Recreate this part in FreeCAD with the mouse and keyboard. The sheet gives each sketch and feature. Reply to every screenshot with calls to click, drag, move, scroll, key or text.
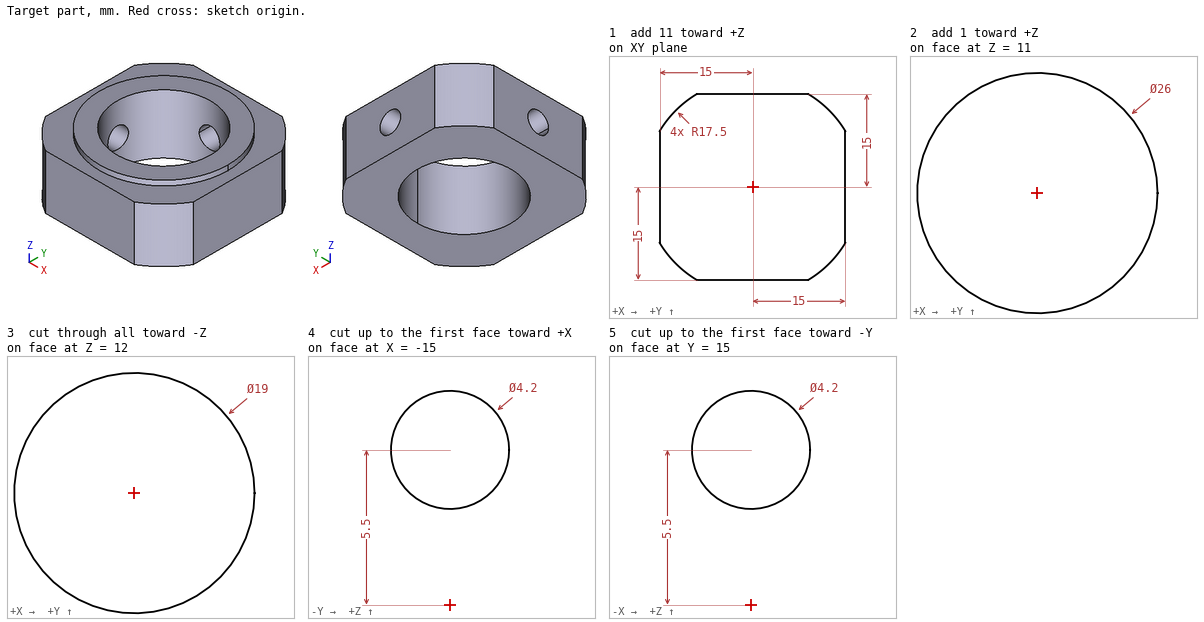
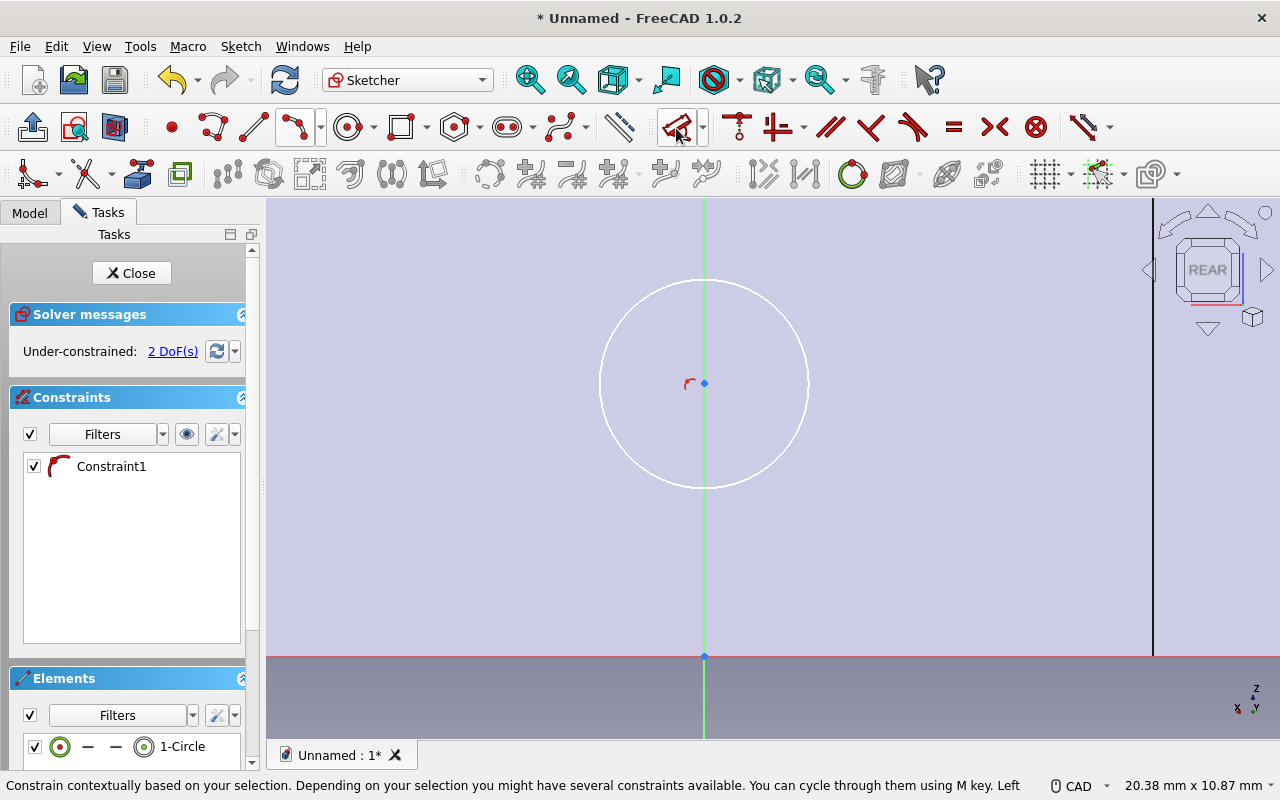
click(778, 310)
click(801, 287)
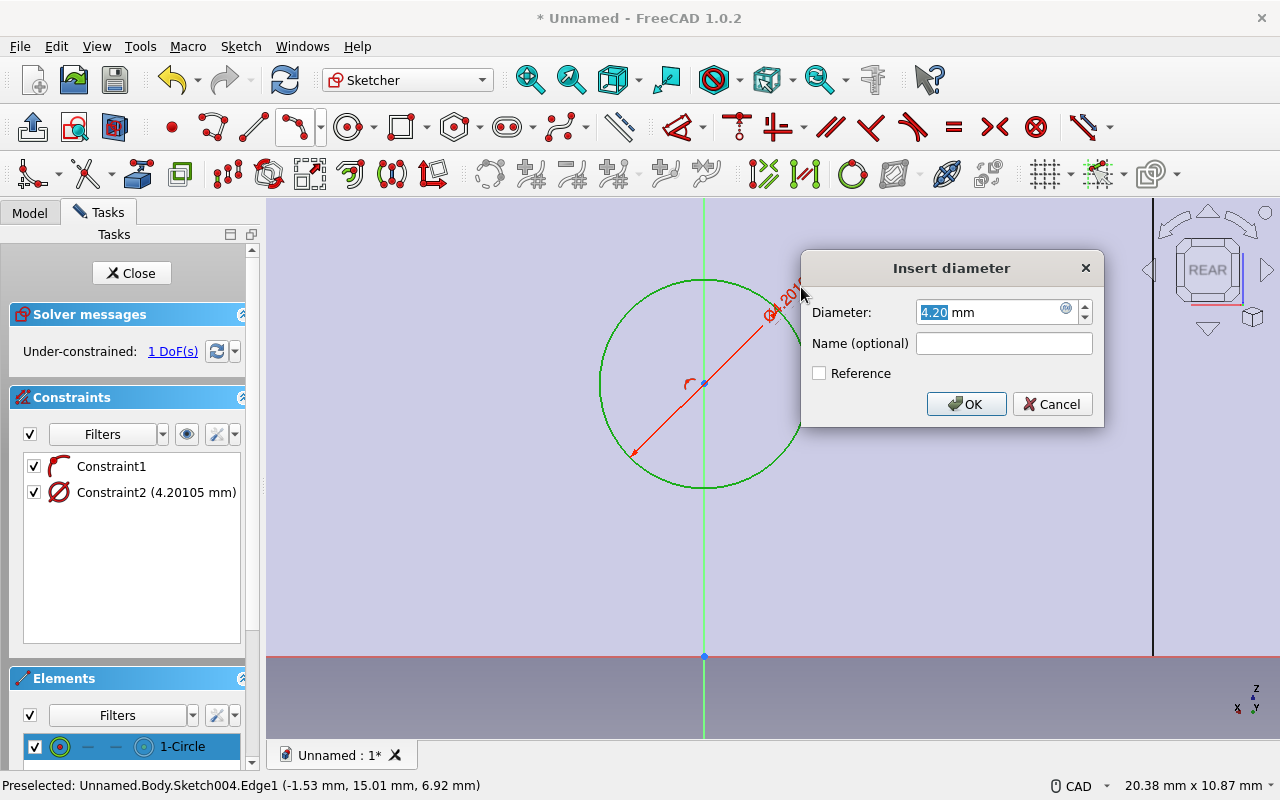
text(4.2)
key(Return)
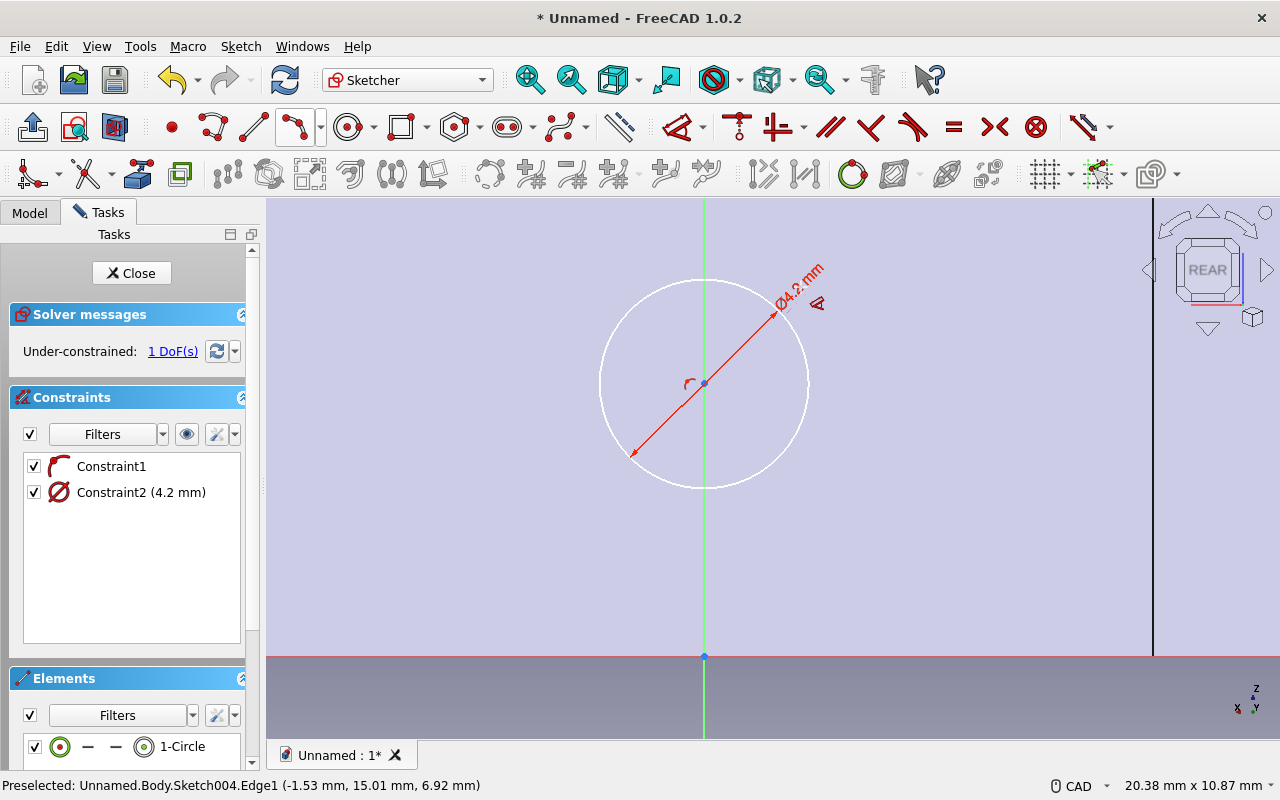
click(704, 384)
click(738, 520)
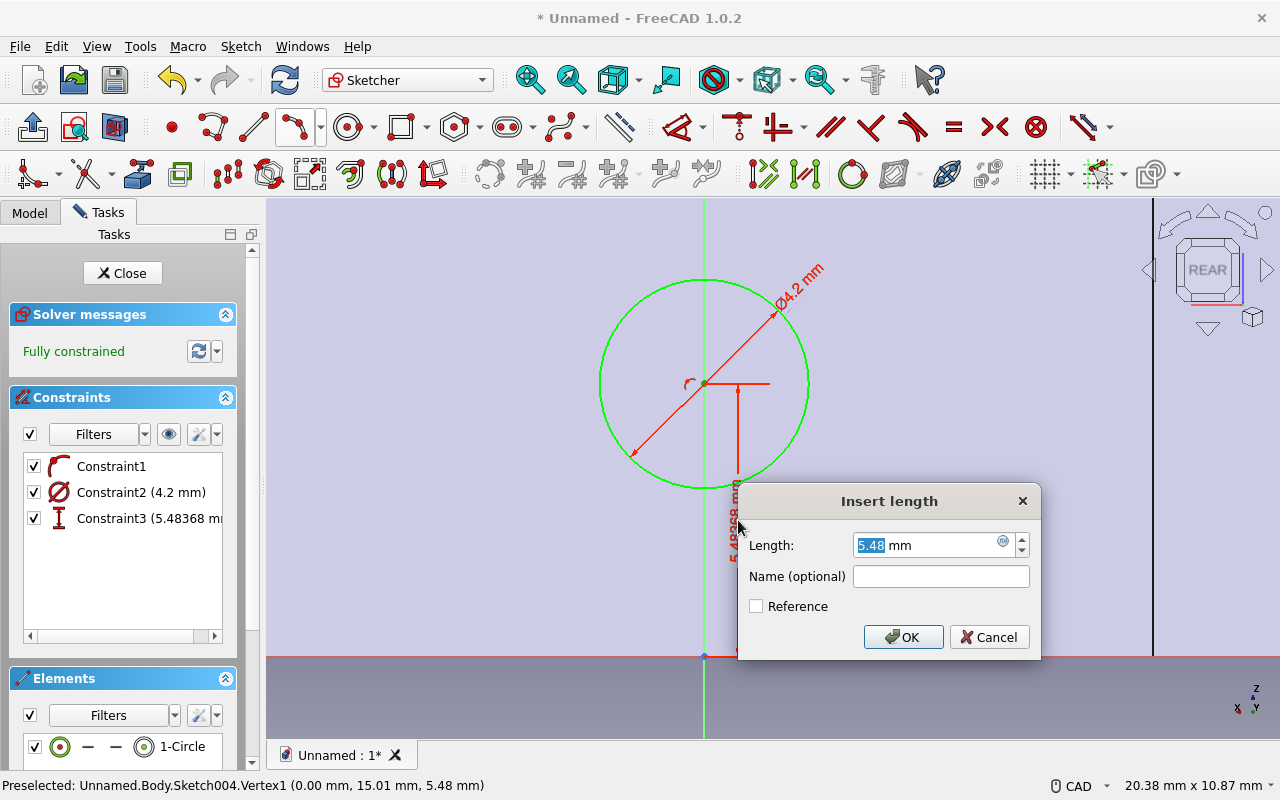
text(5.5)
key(Return)
key(Escape)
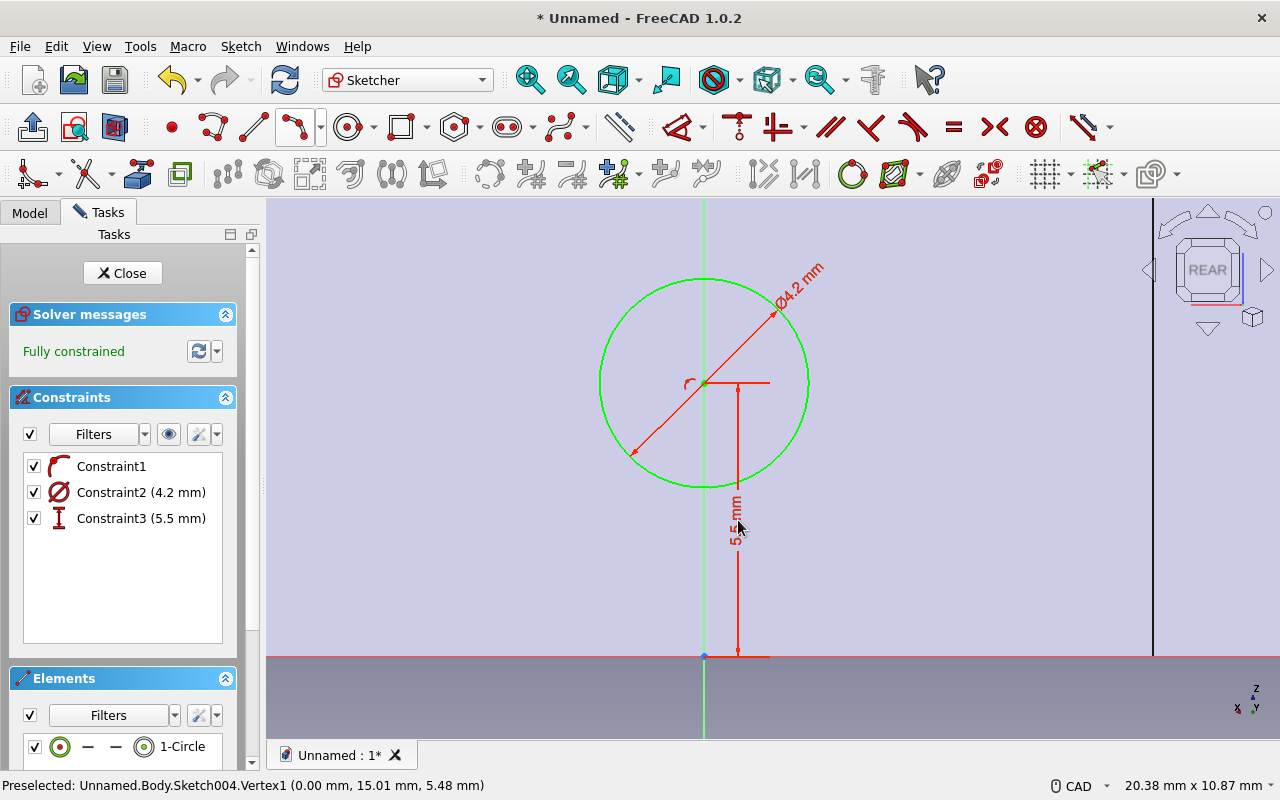
click(123, 273)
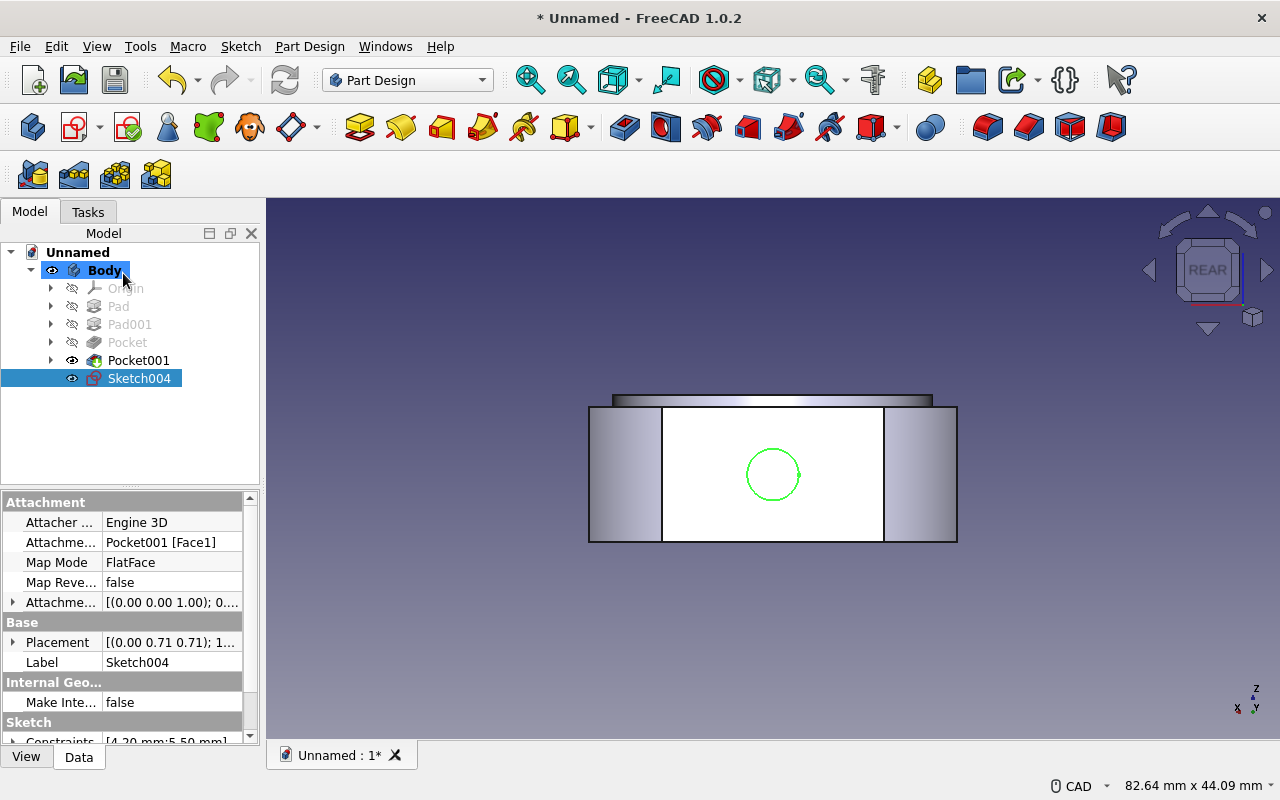
click(625, 128)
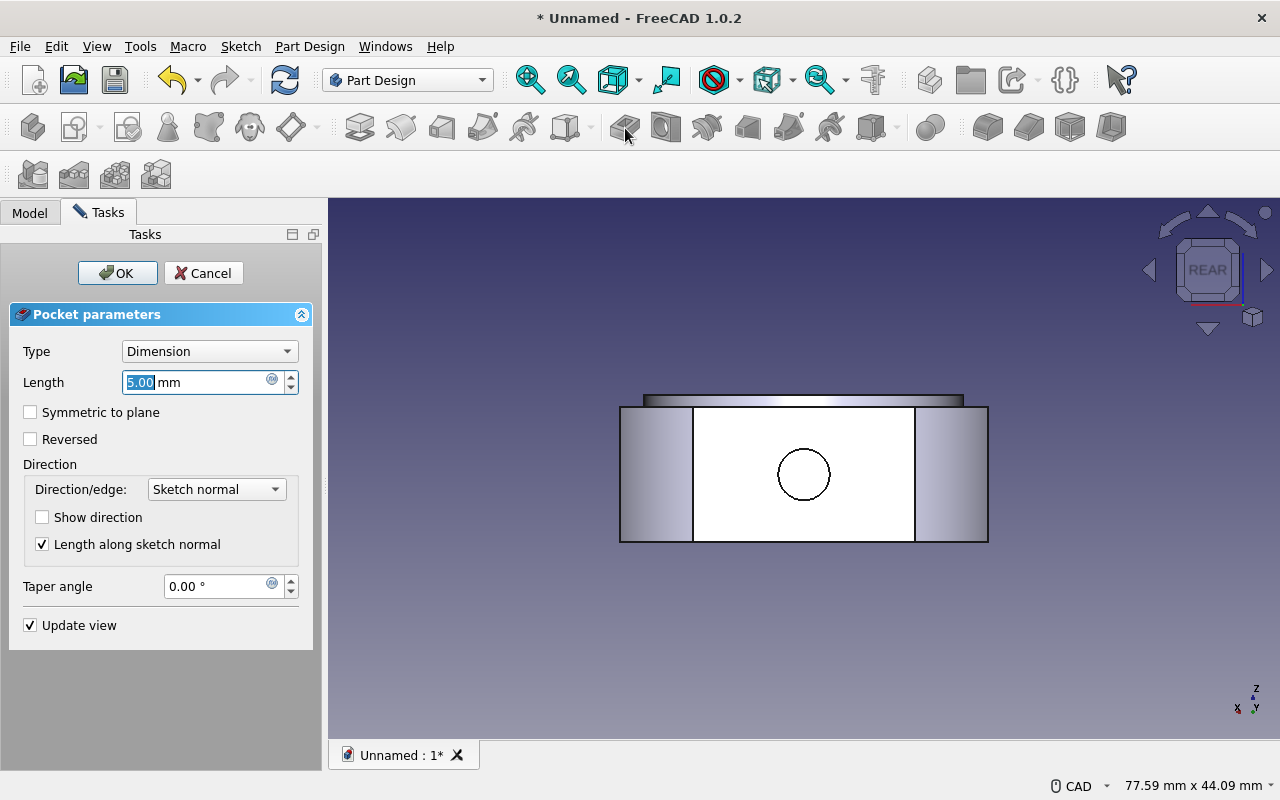
click(210, 352)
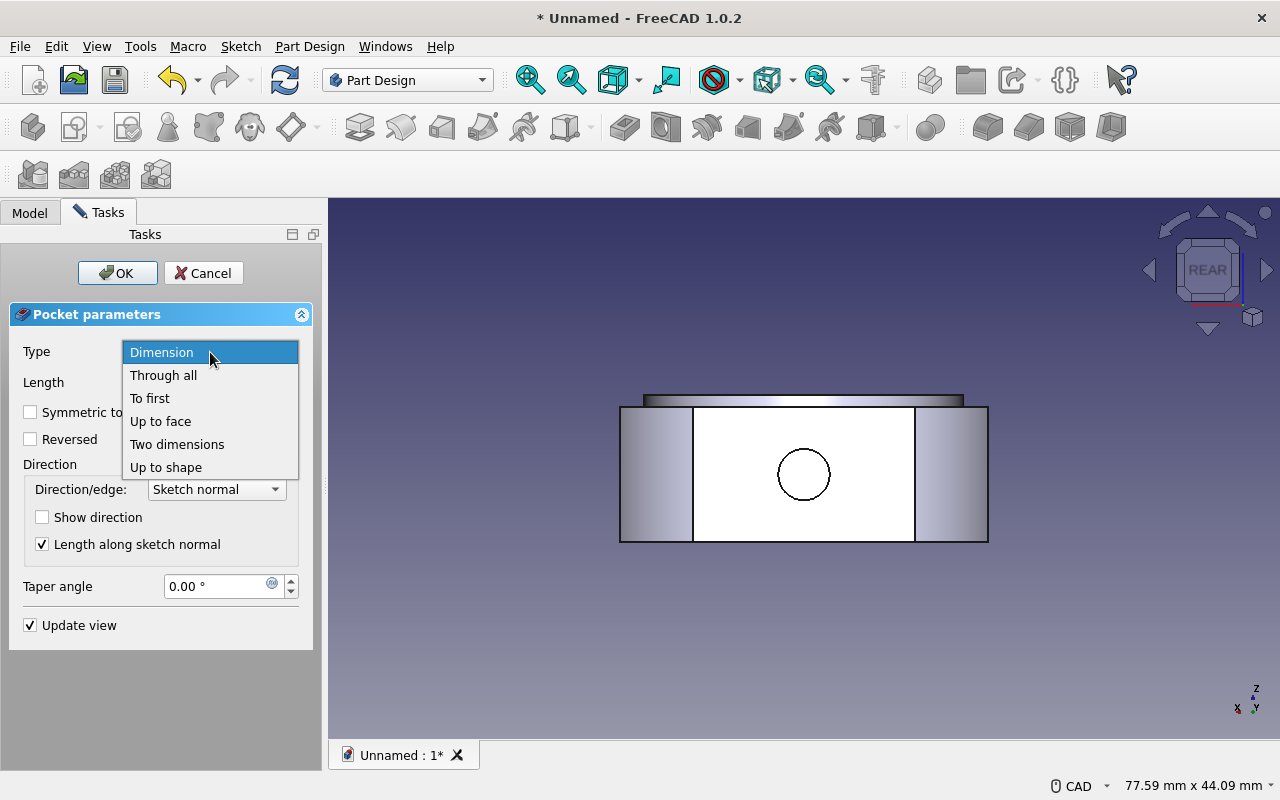
click(208, 398)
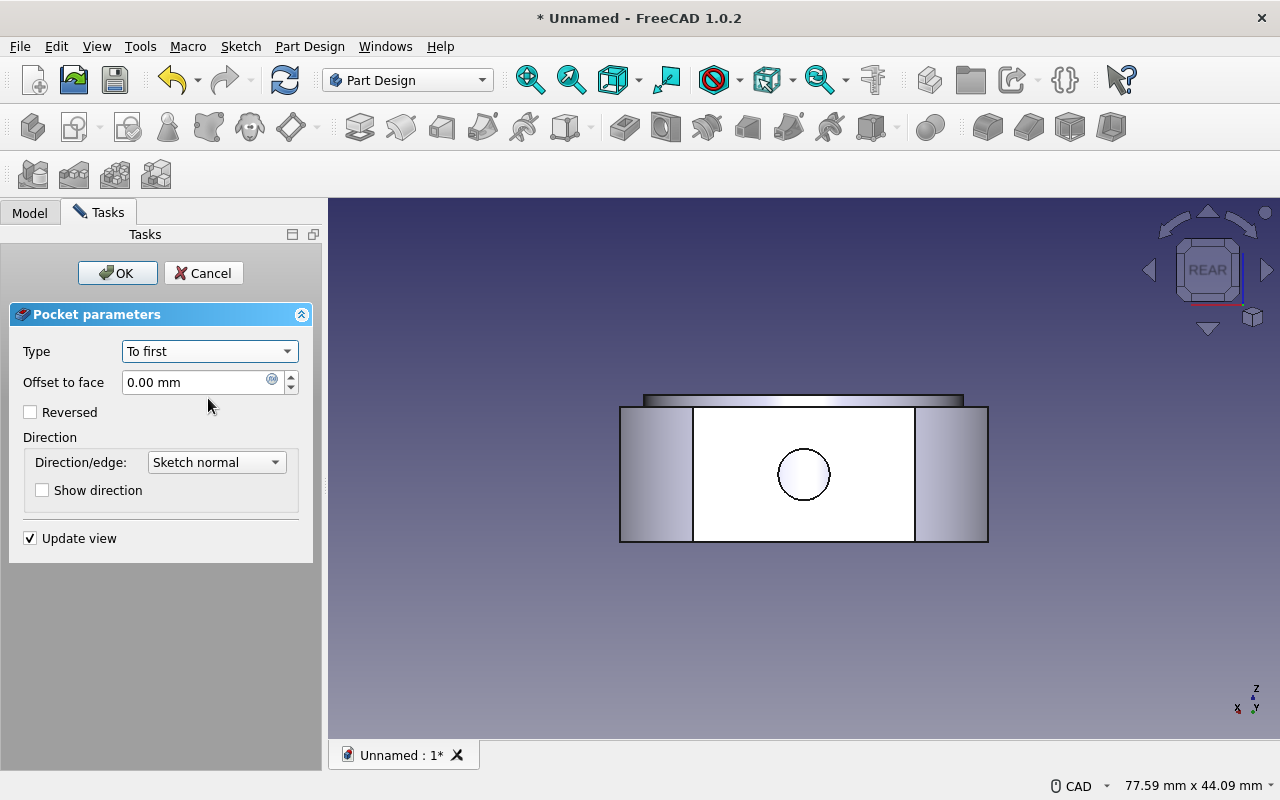
click(118, 273)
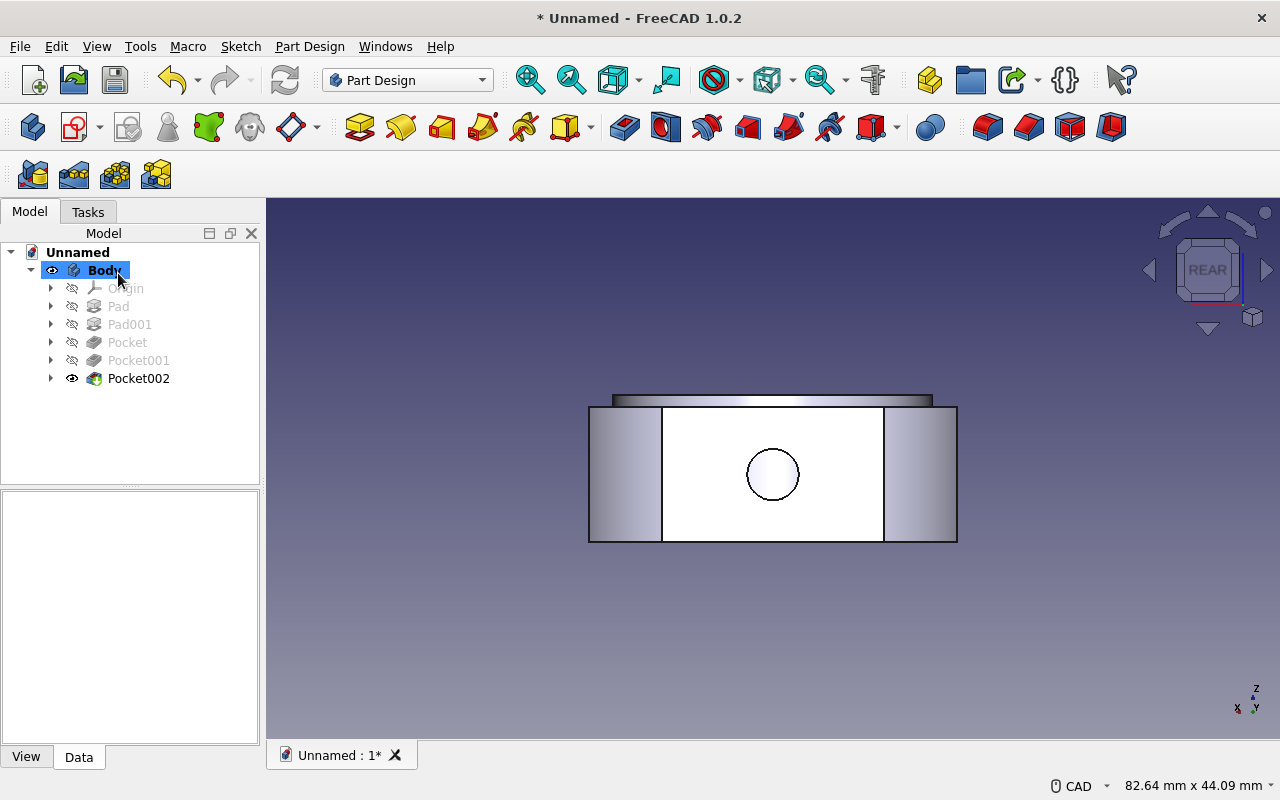
key(0)